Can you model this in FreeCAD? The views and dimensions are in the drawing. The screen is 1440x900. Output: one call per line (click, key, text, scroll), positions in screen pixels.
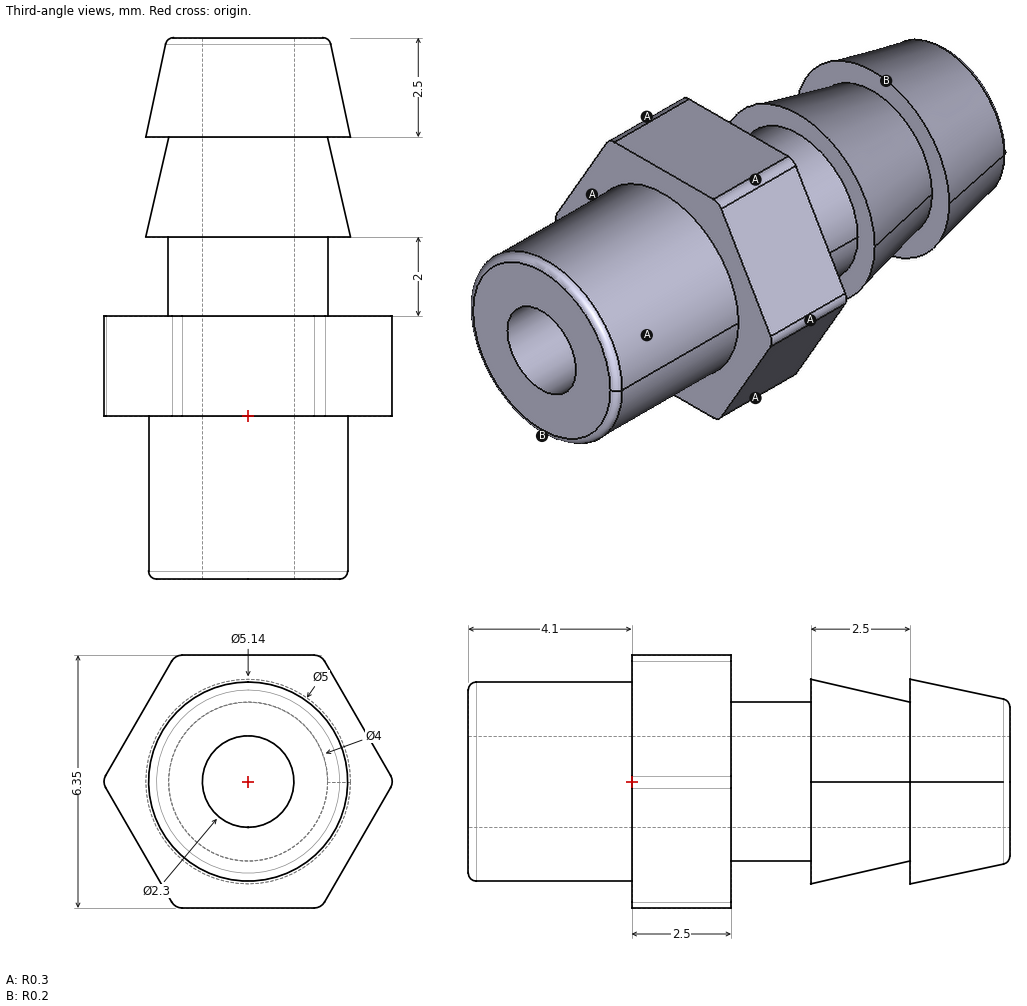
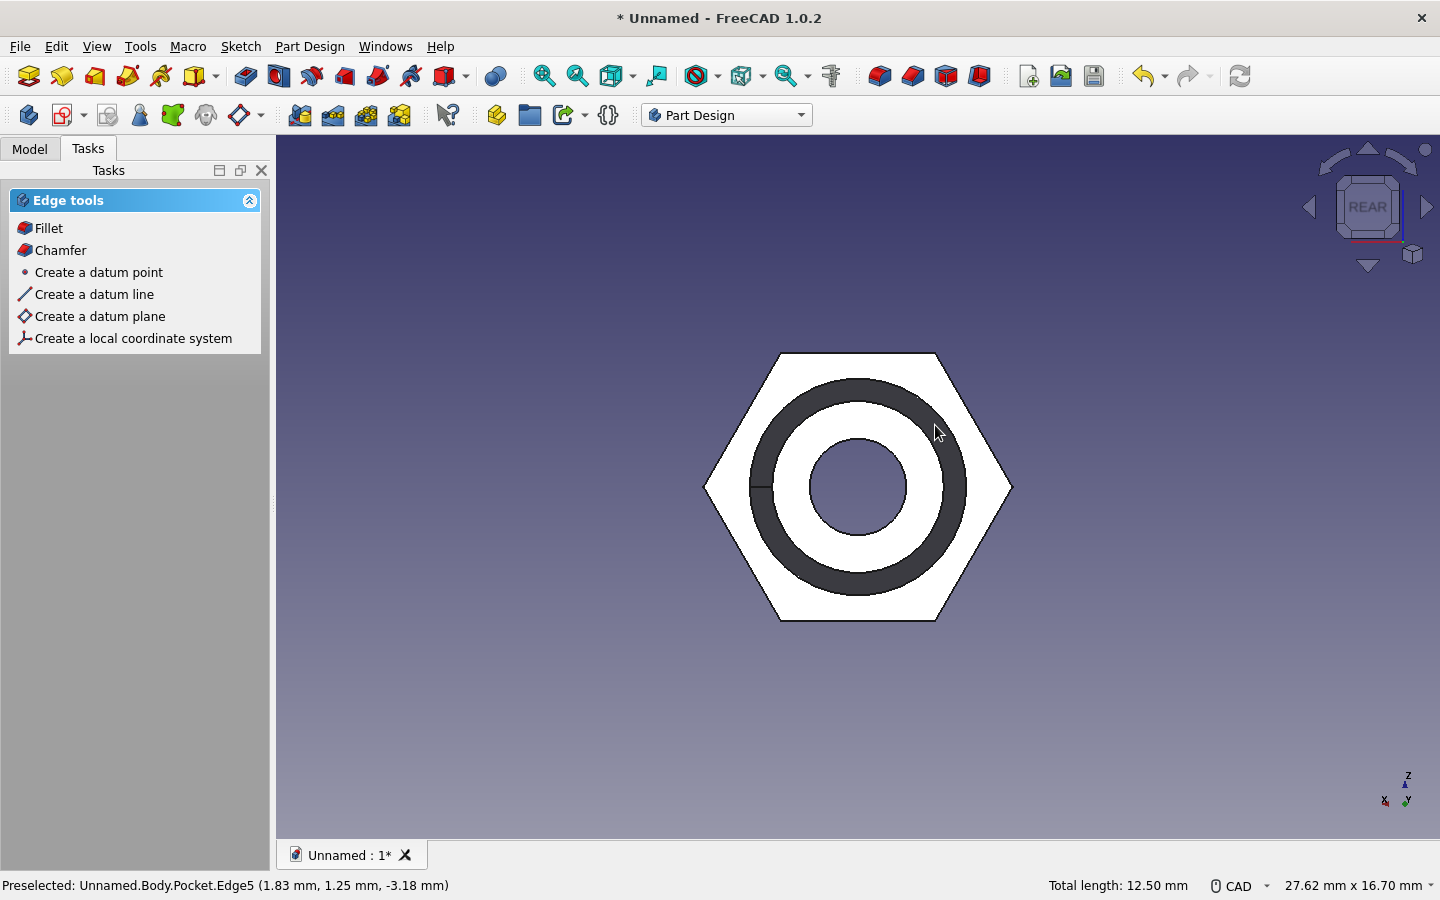
click(545, 76)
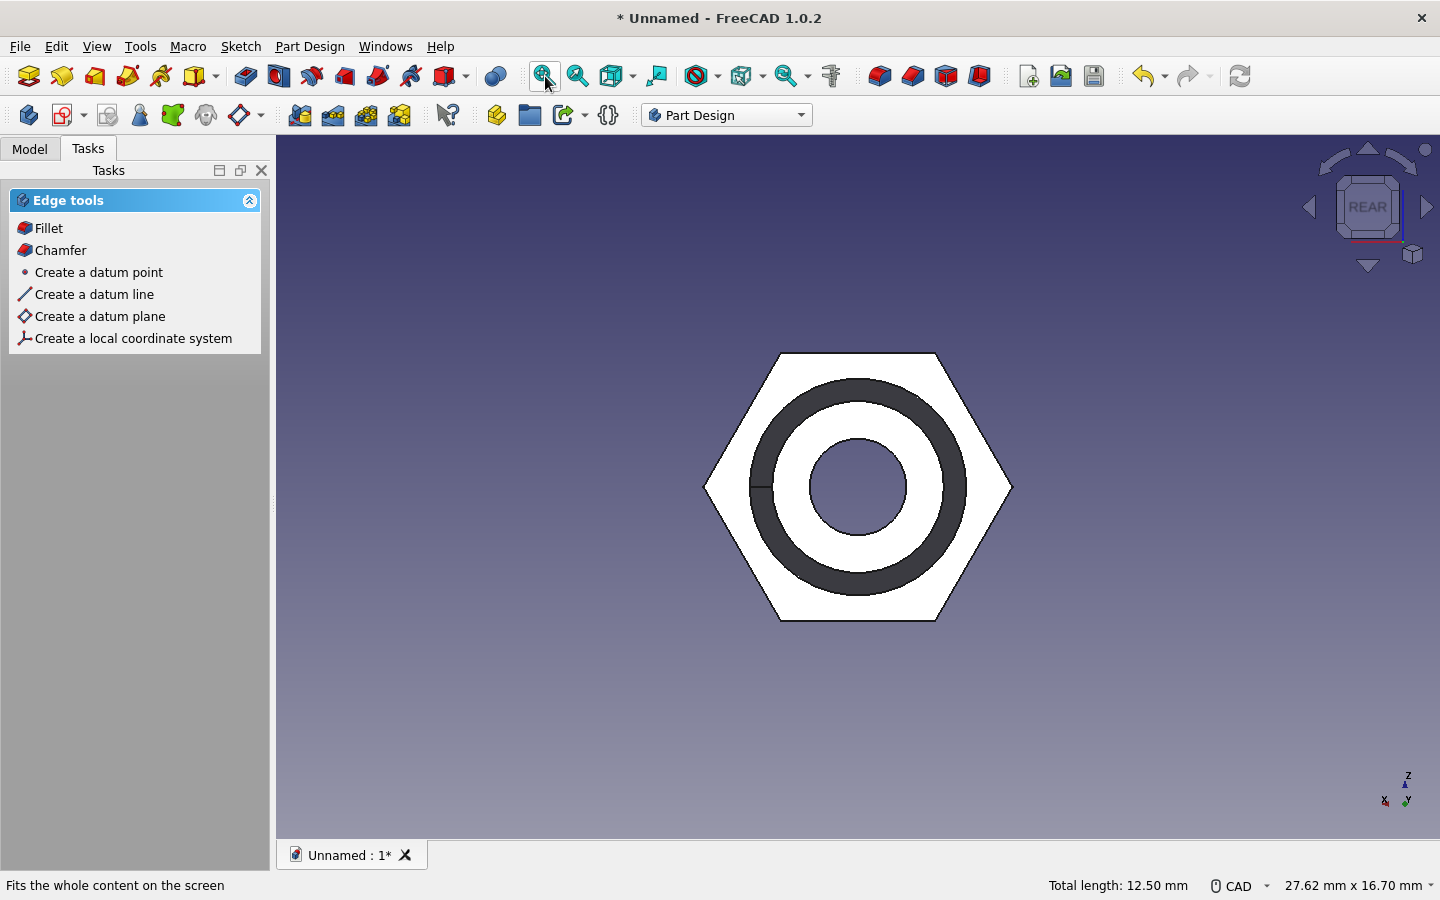
key(6)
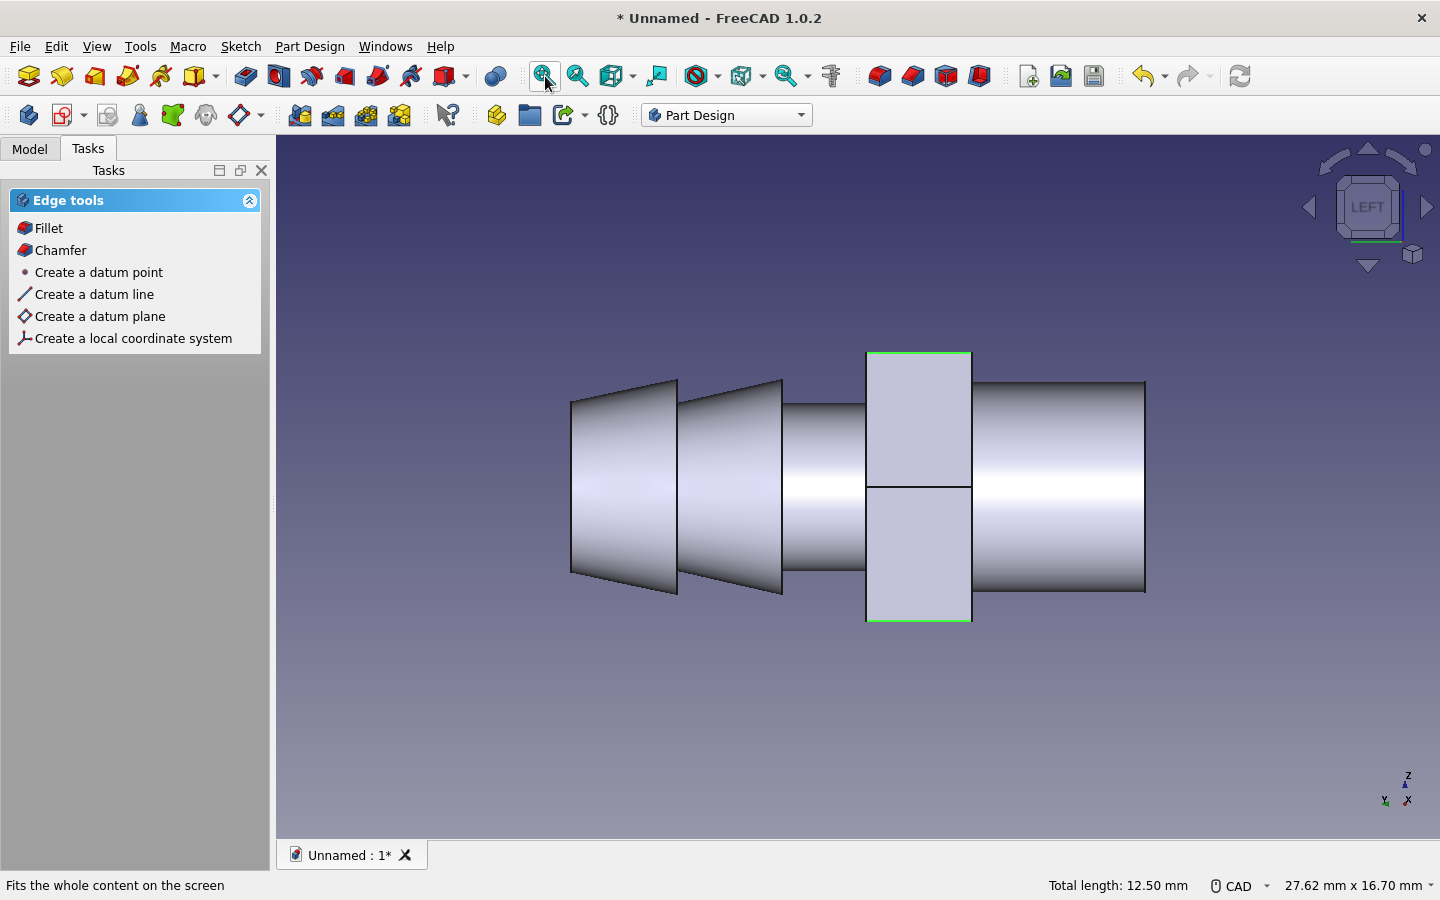
click(919, 486, ctrl)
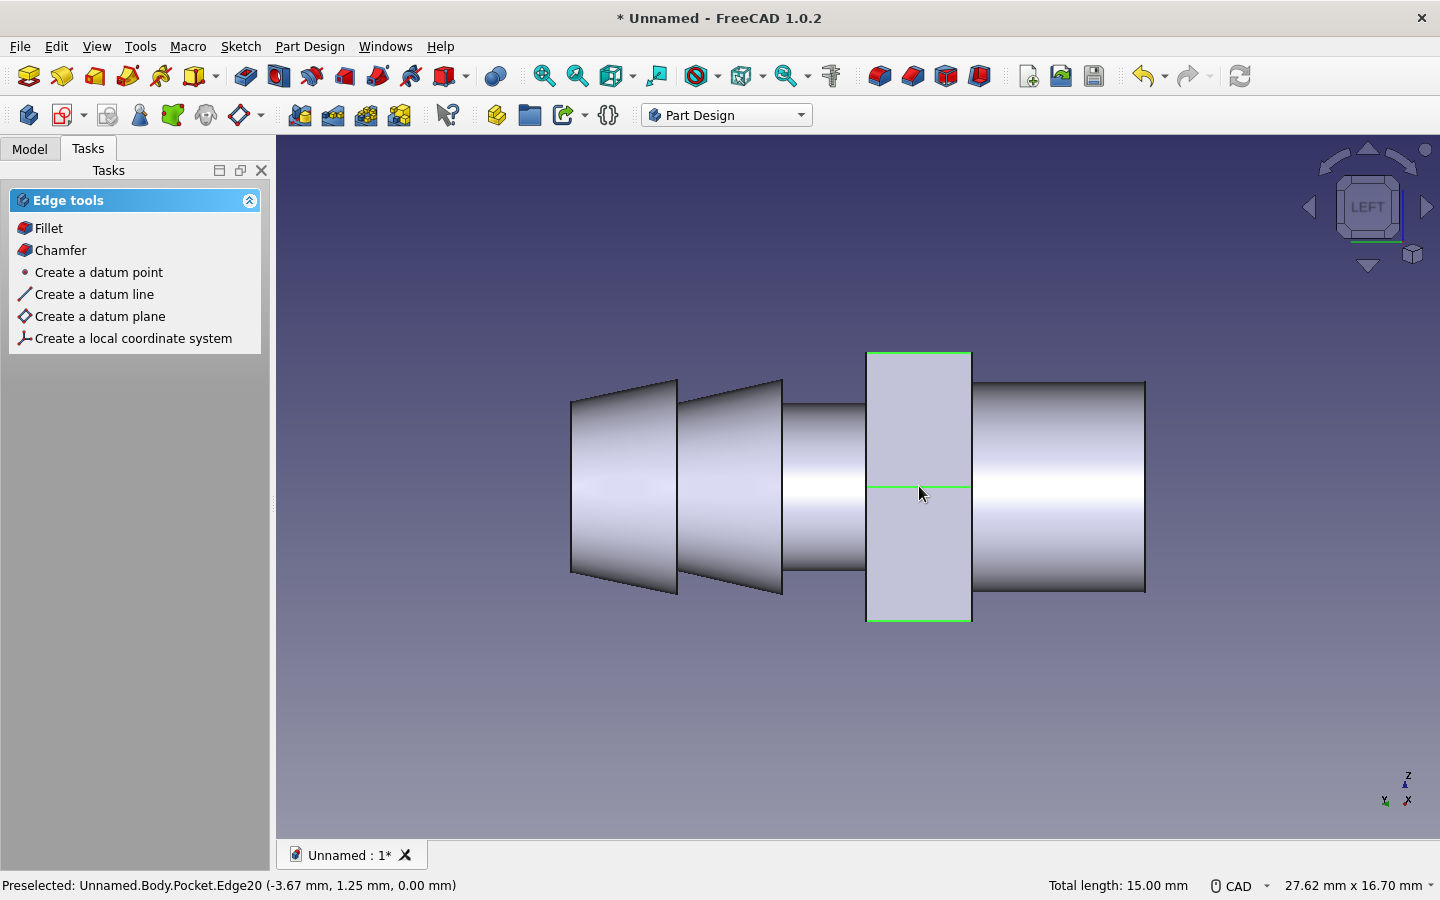
click(880, 76)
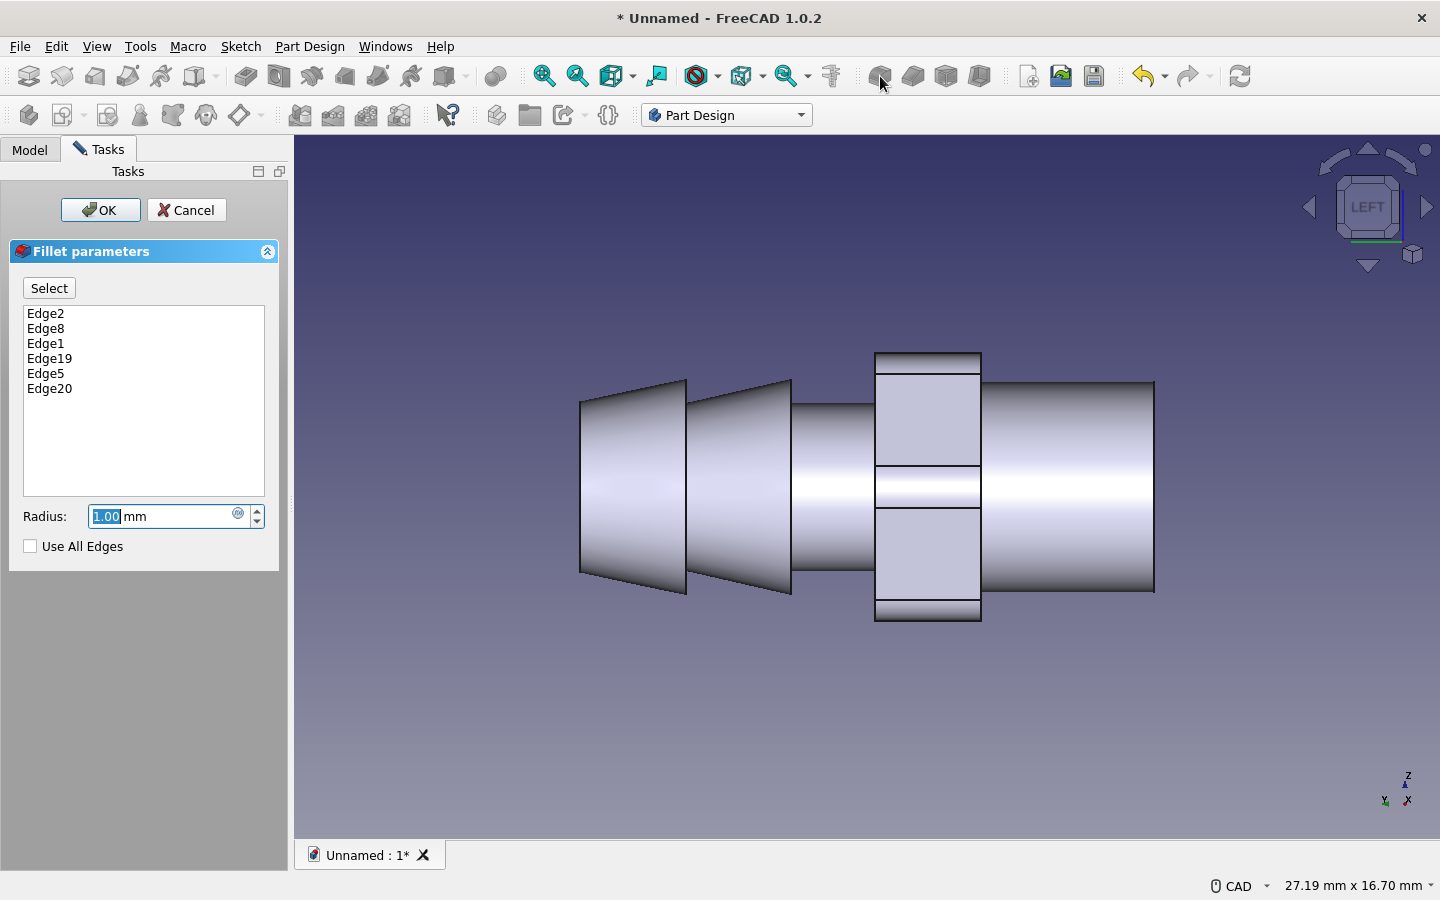
text(0.3)
key(Tab)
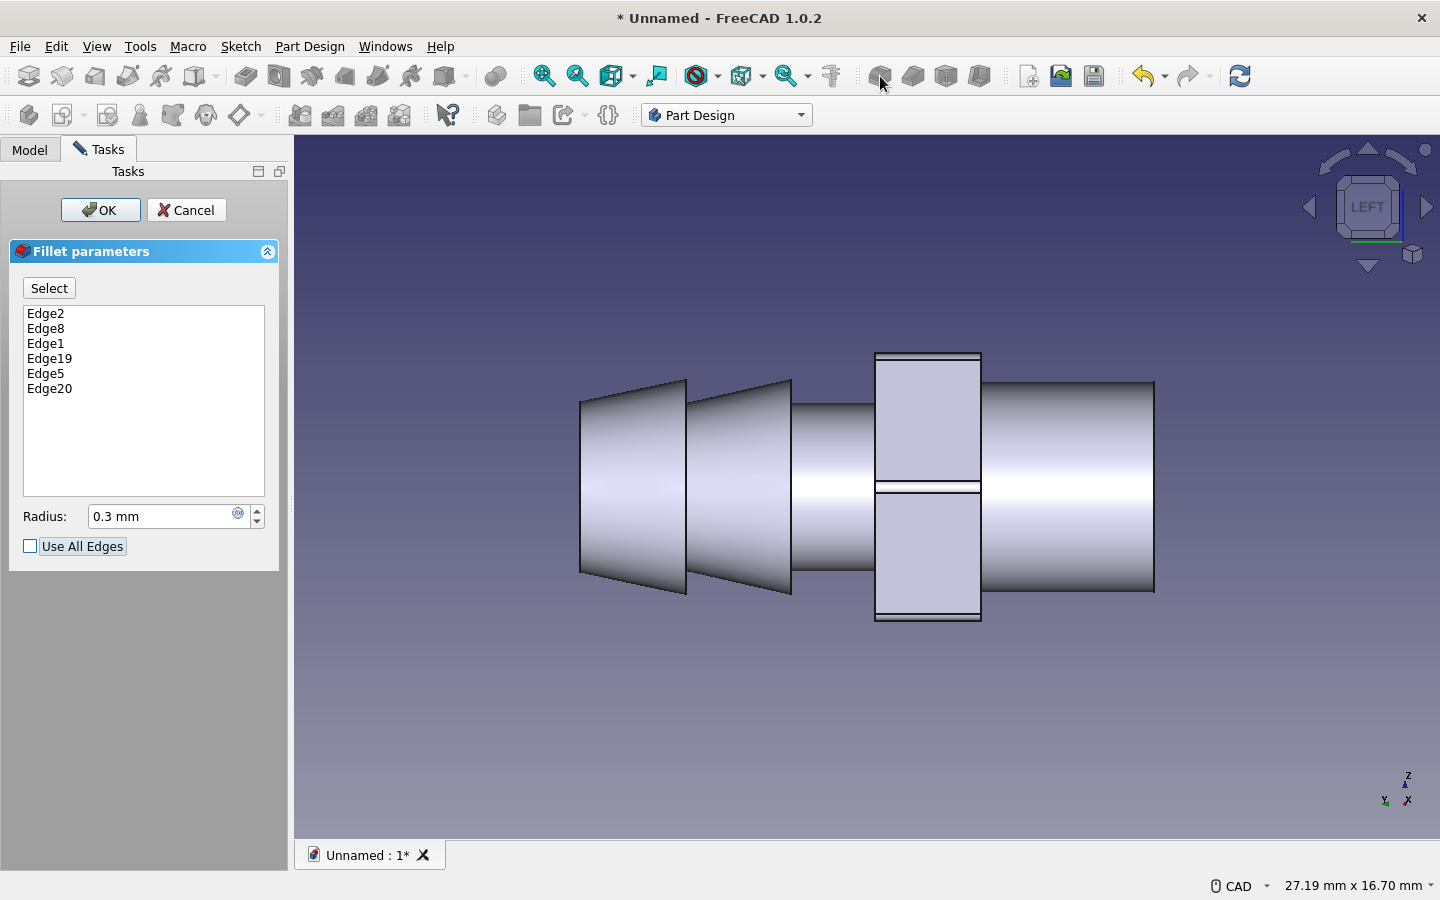
click(101, 210)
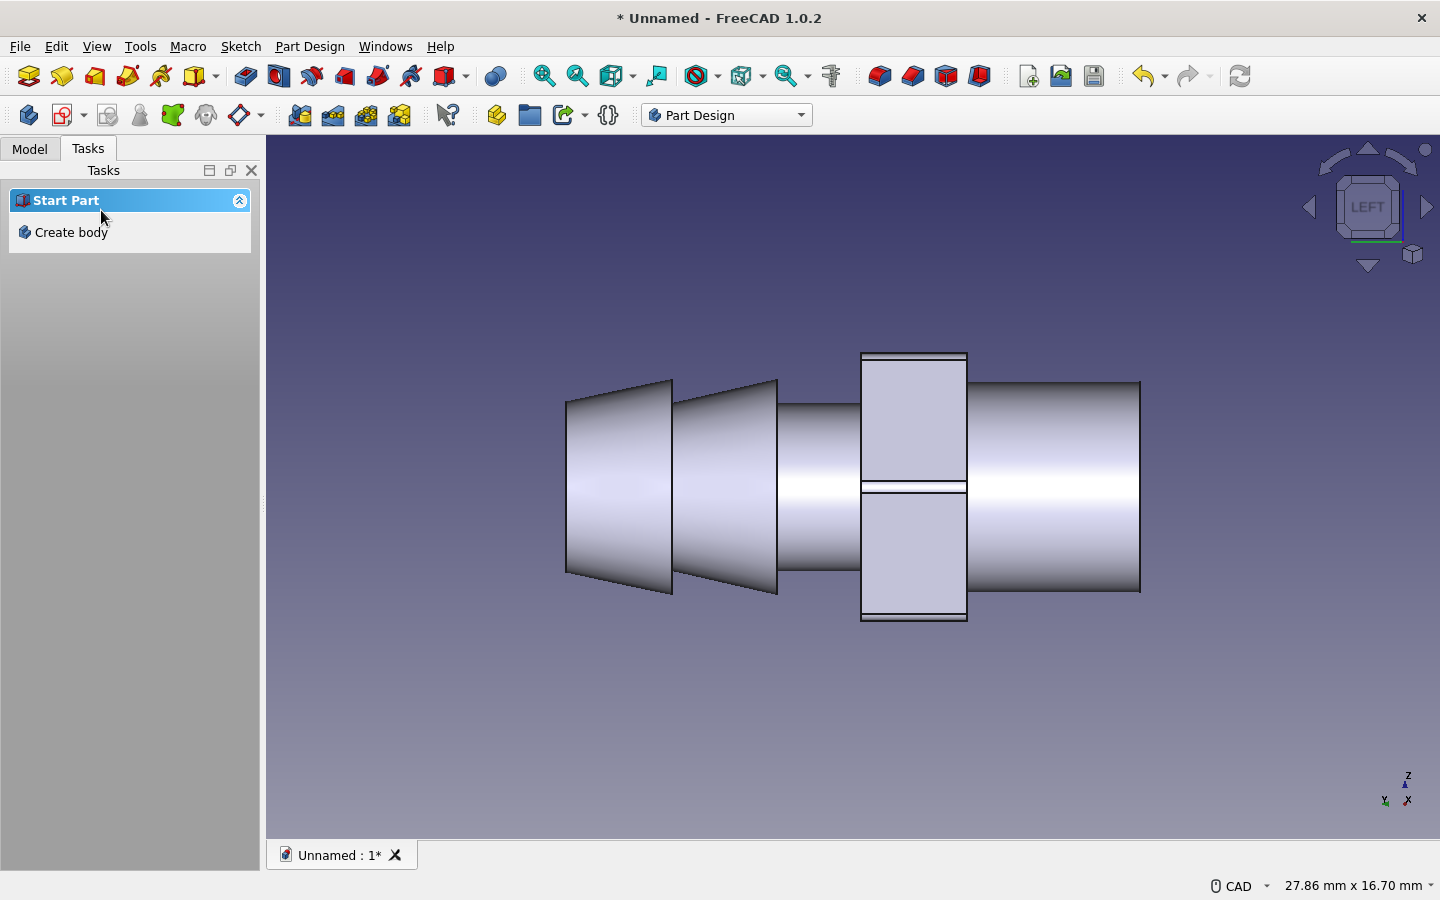
click(1140, 486)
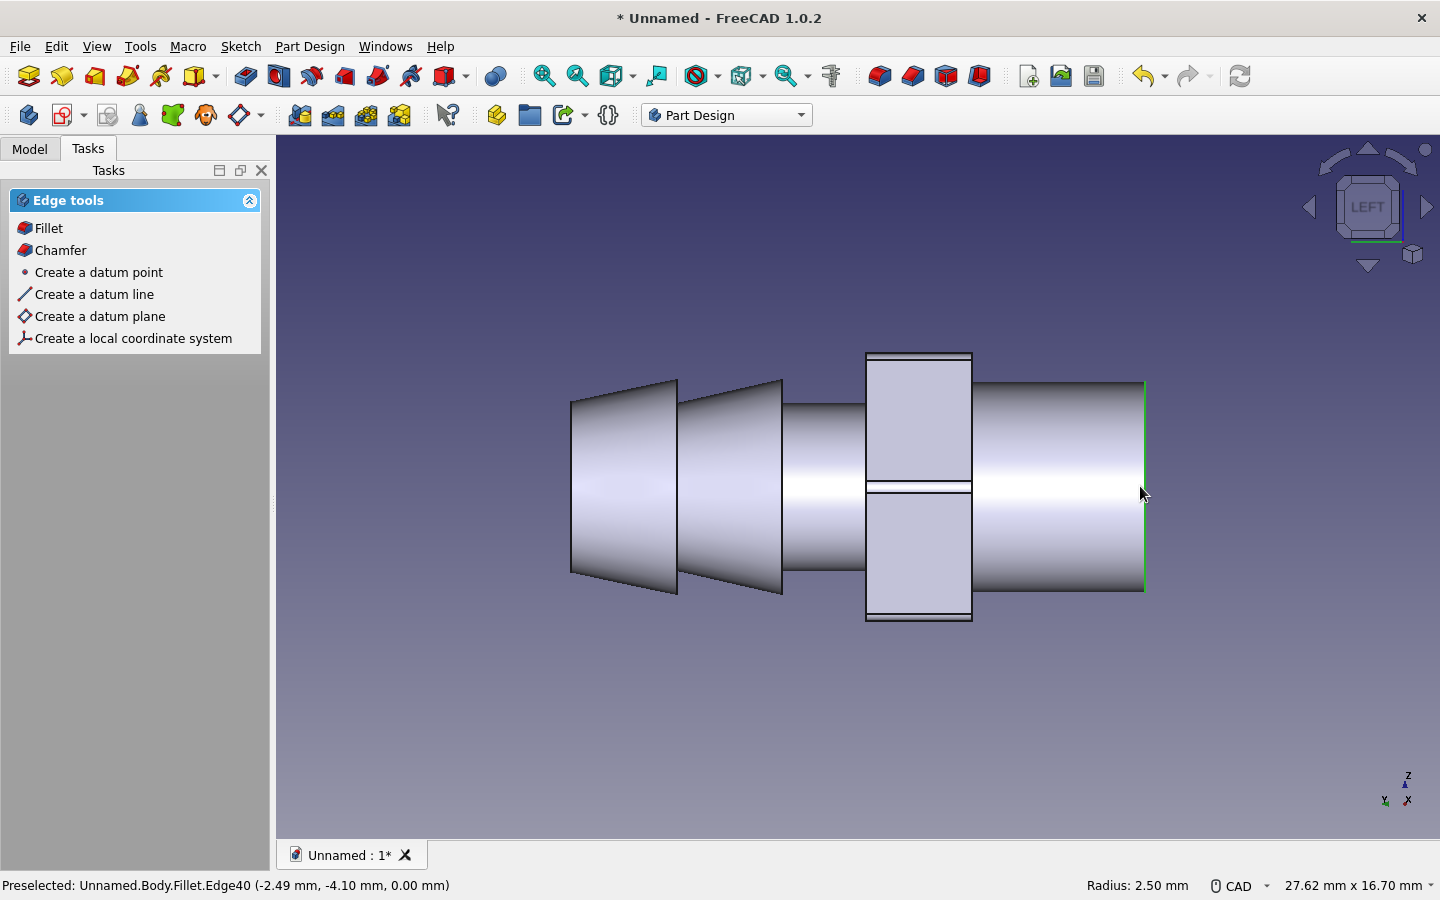
key(0)